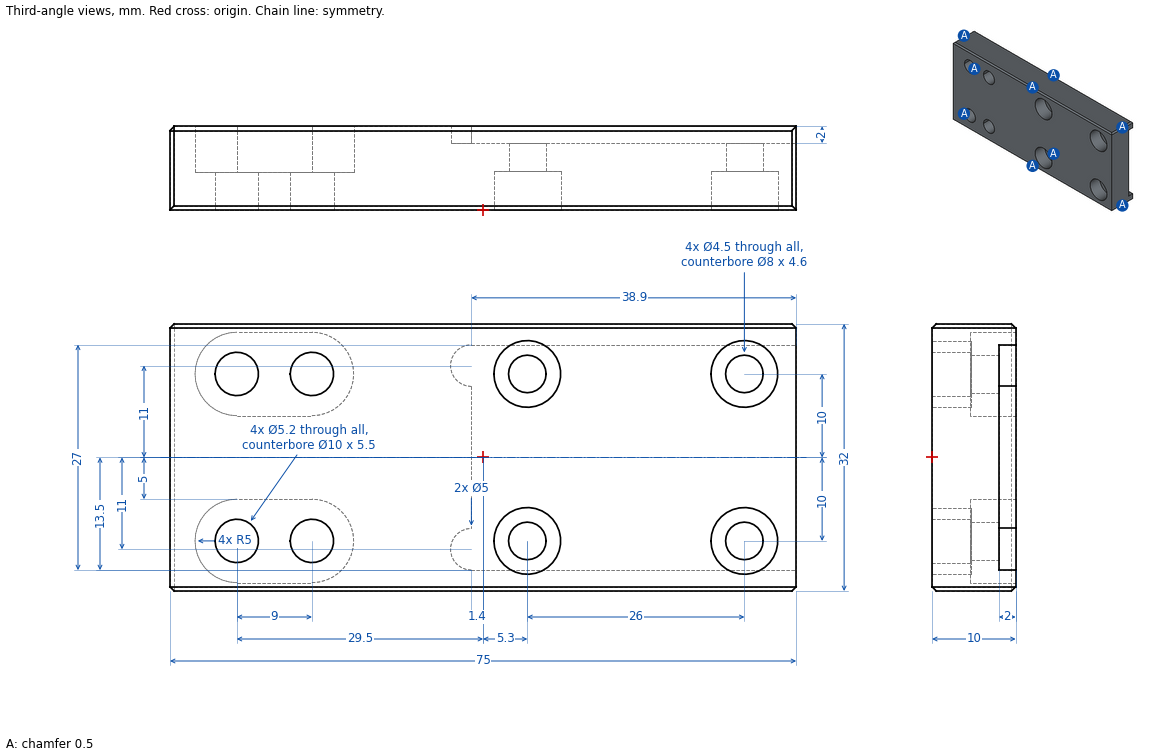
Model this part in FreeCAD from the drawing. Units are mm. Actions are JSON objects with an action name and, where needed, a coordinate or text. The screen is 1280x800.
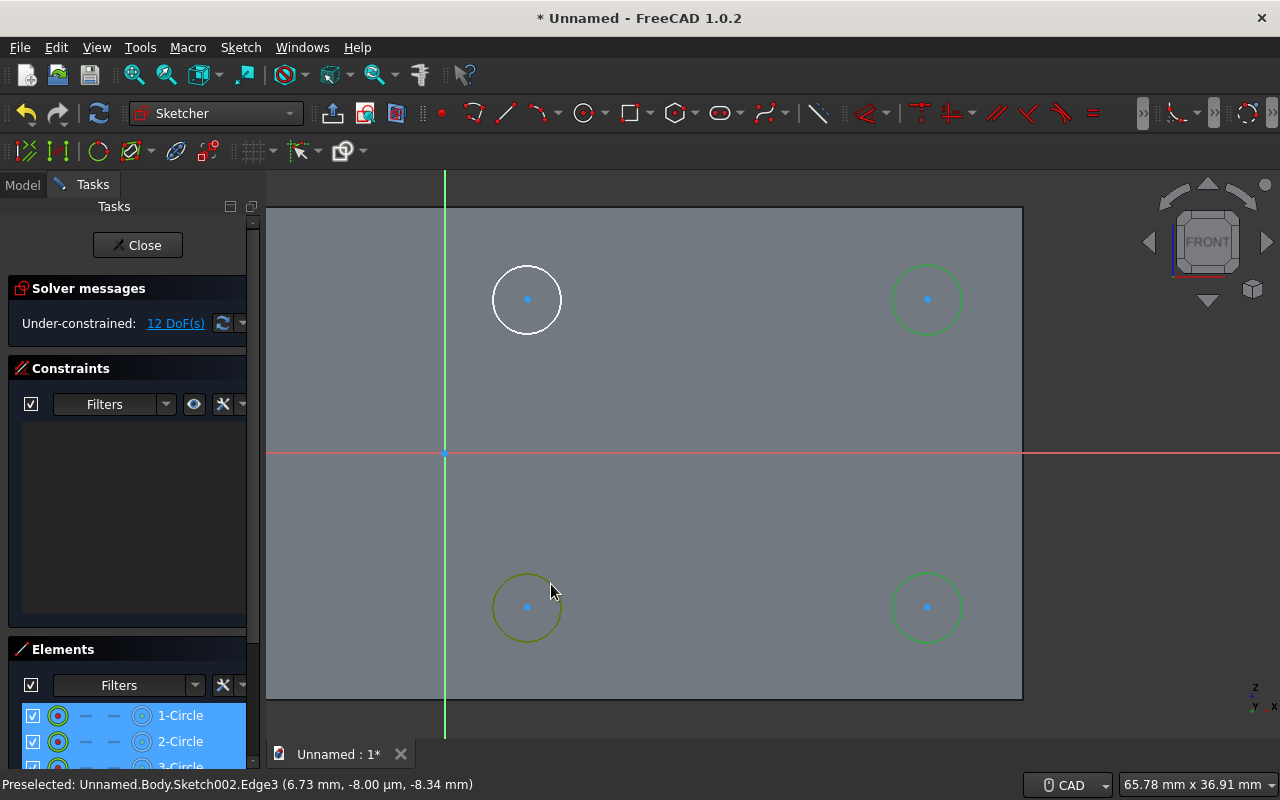
{"action": "left_click", "coordinate": [551, 276]}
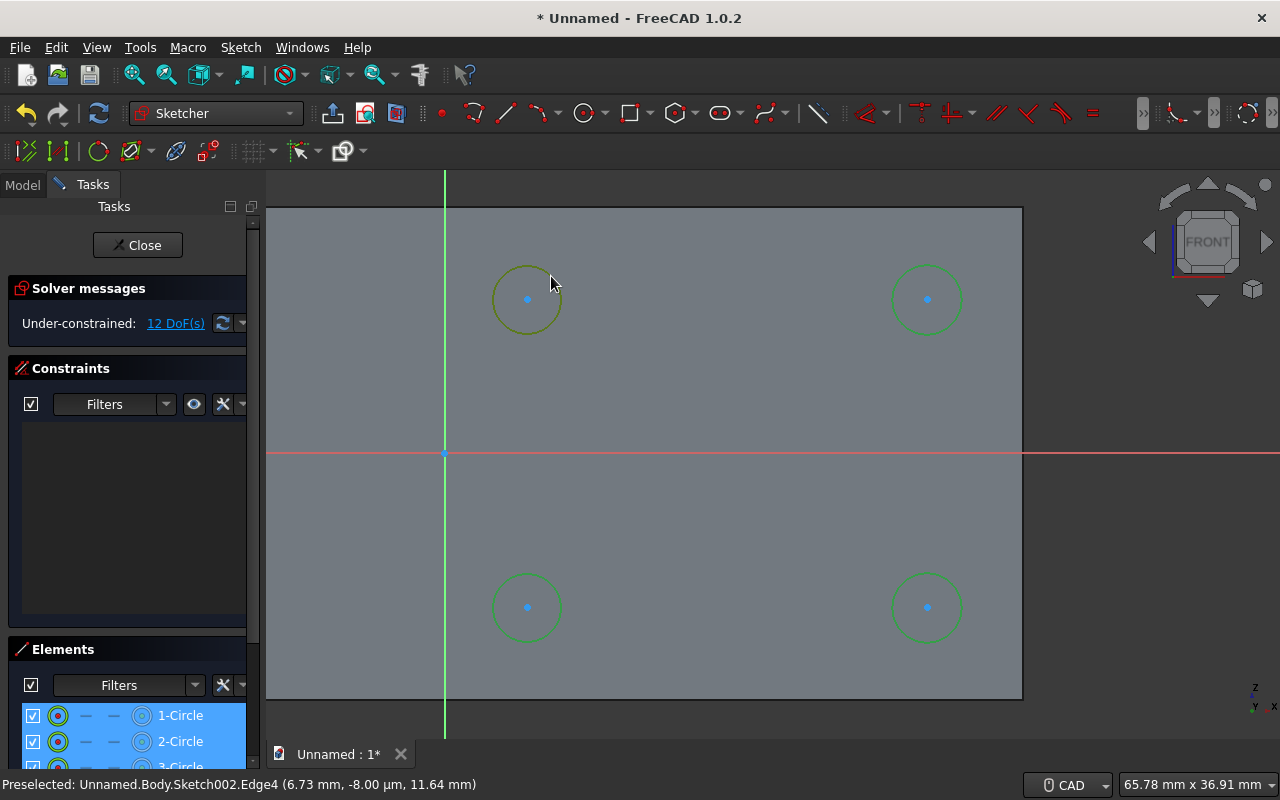
{"action": "left_click", "coordinate": [1094, 114]}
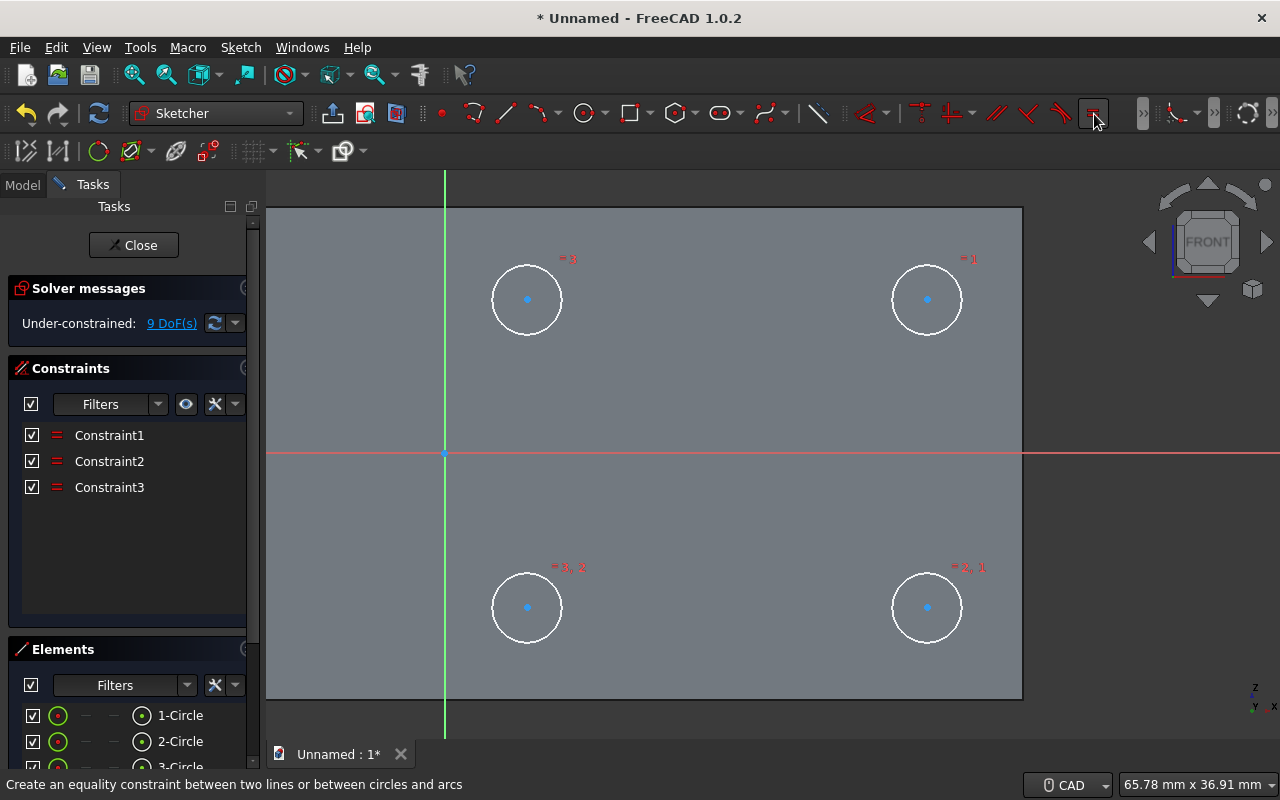
{"action": "left_click", "coordinate": [927, 300]}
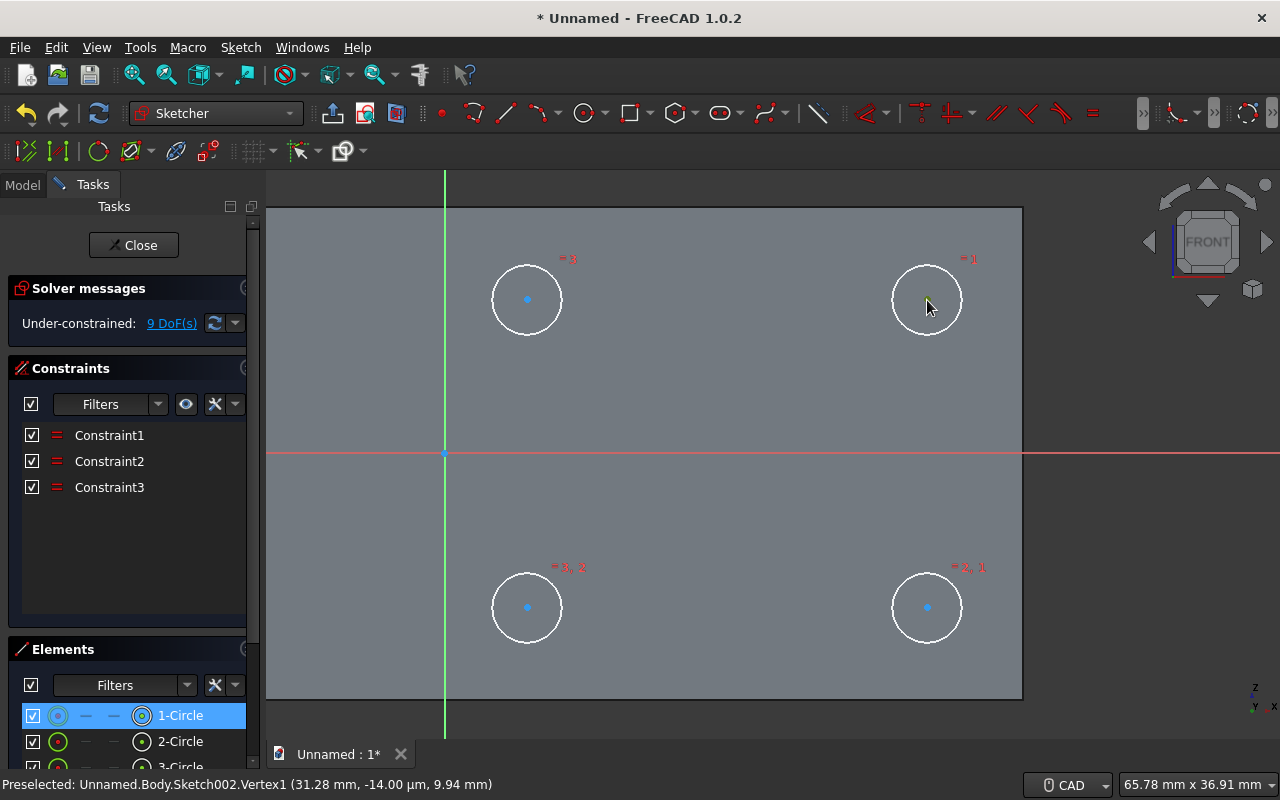
{"action": "left_click", "coordinate": [927, 608]}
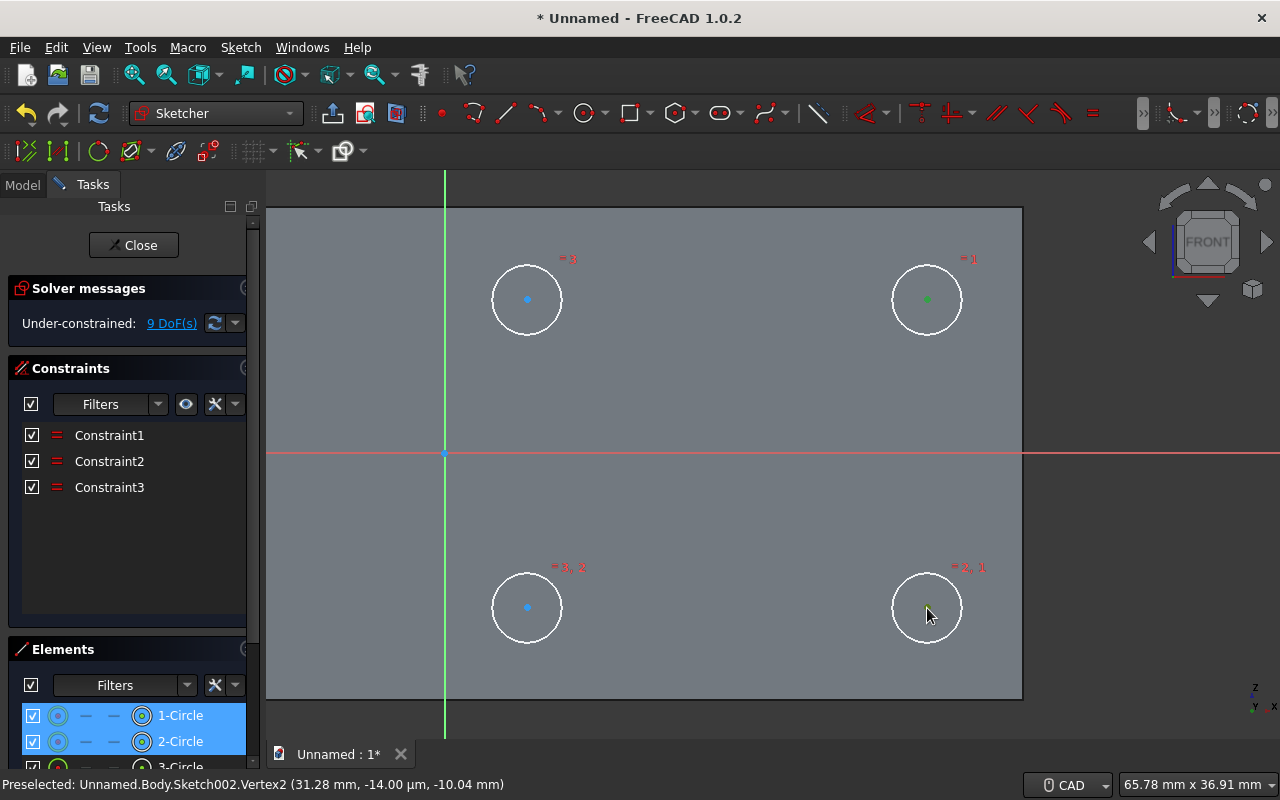
{"action": "left_click", "coordinate": [974, 114]}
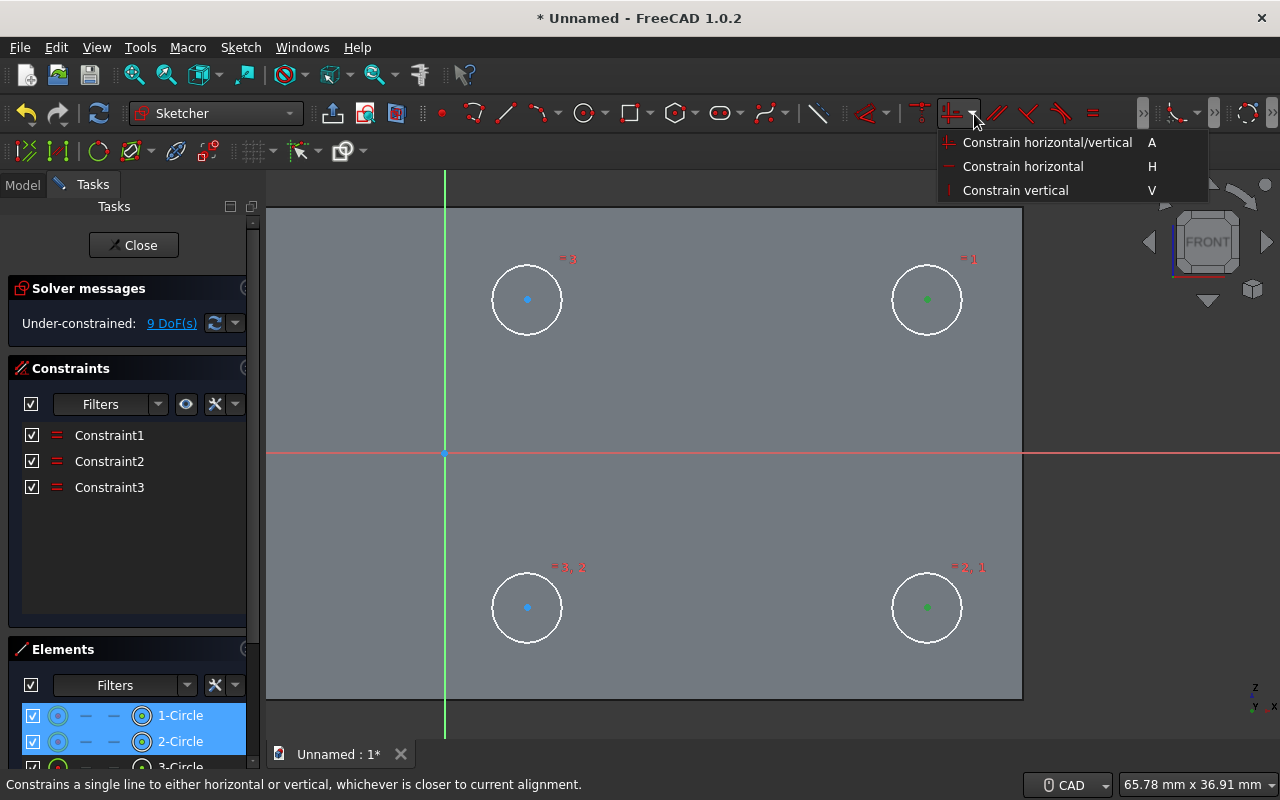
{"action": "left_click", "coordinate": [1073, 190]}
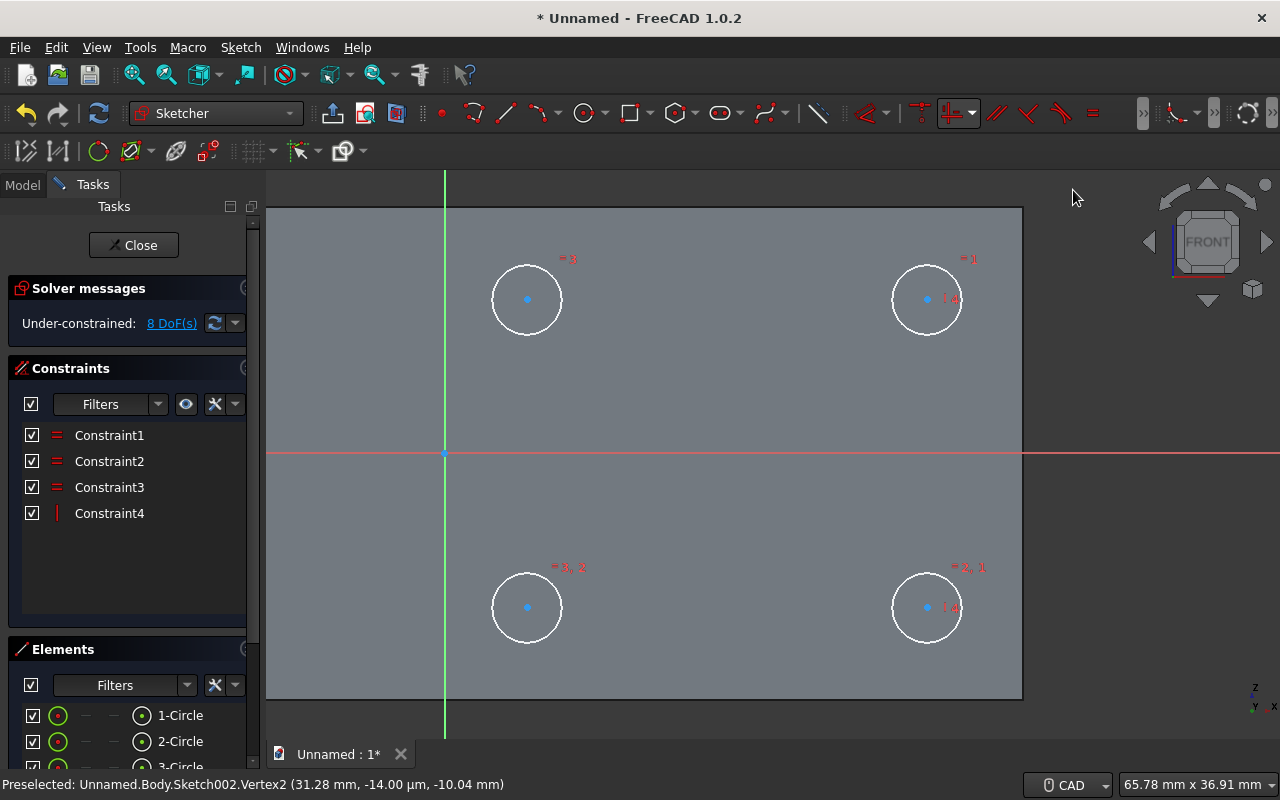
{"action": "left_click", "coordinate": [927, 608]}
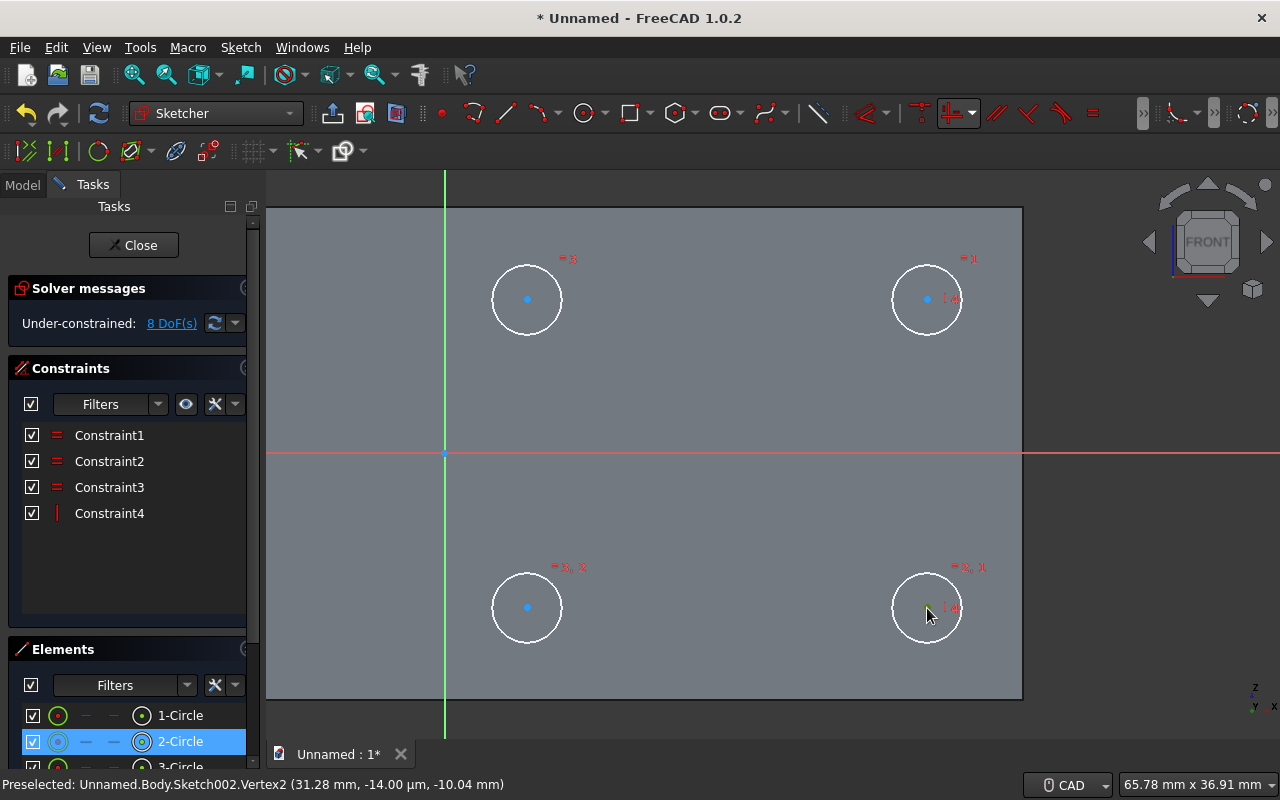
{"action": "left_click", "coordinate": [527, 608]}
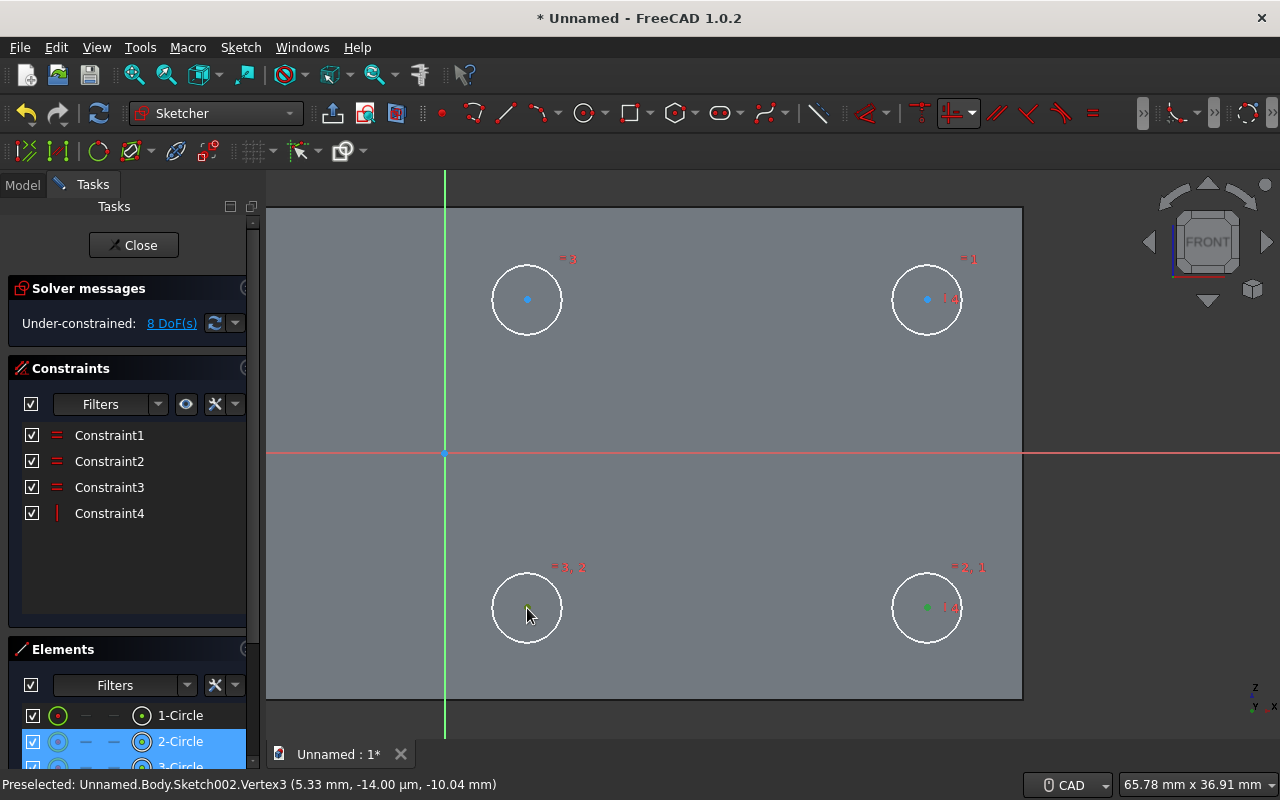
{"action": "left_click", "coordinate": [974, 114]}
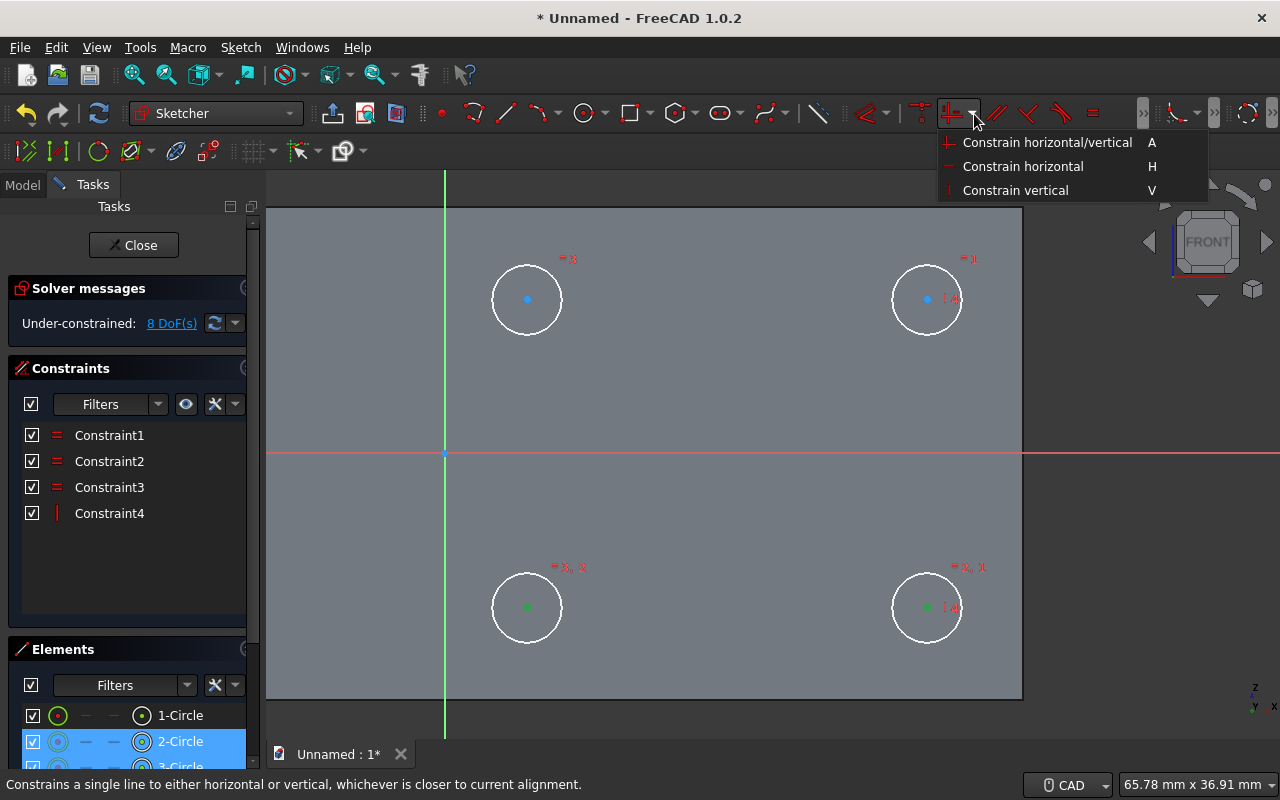
{"action": "left_click", "coordinate": [1073, 166]}